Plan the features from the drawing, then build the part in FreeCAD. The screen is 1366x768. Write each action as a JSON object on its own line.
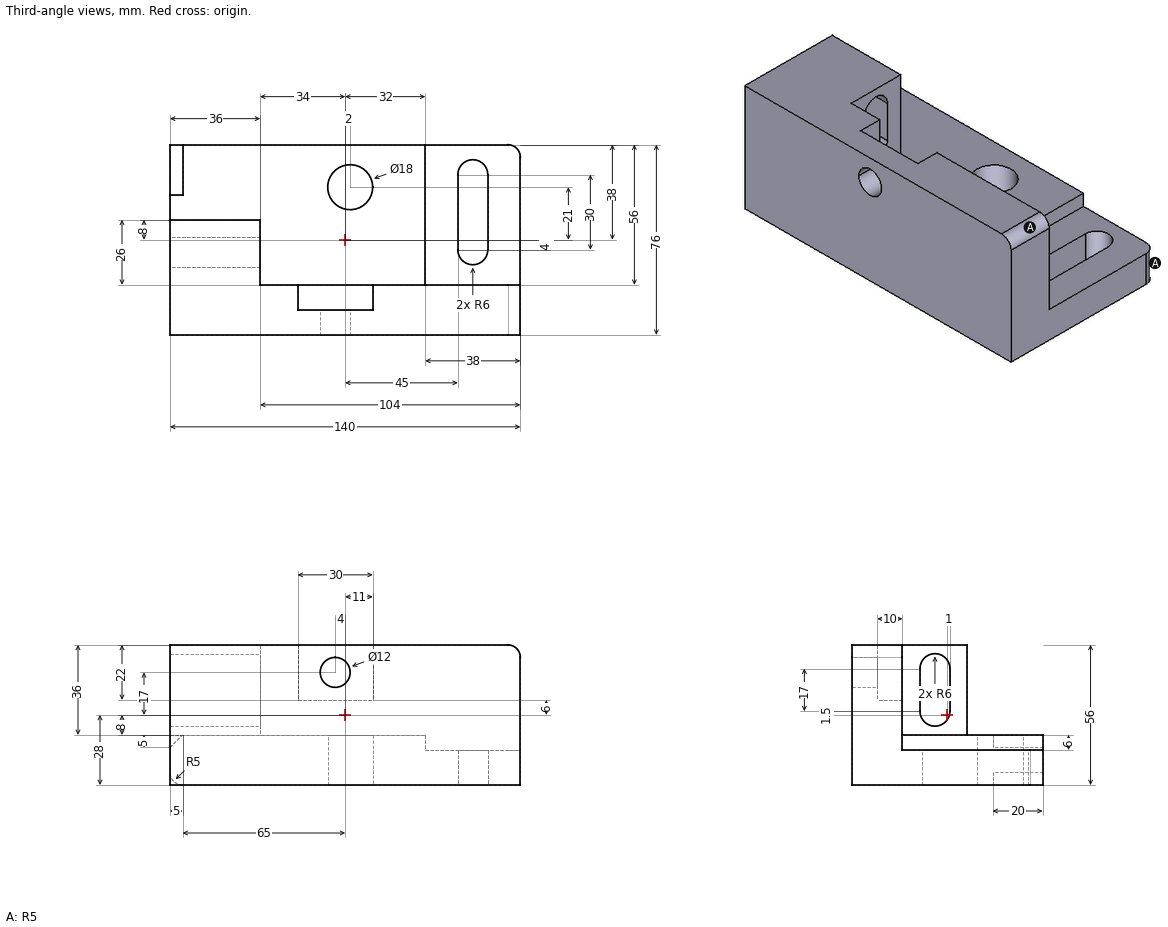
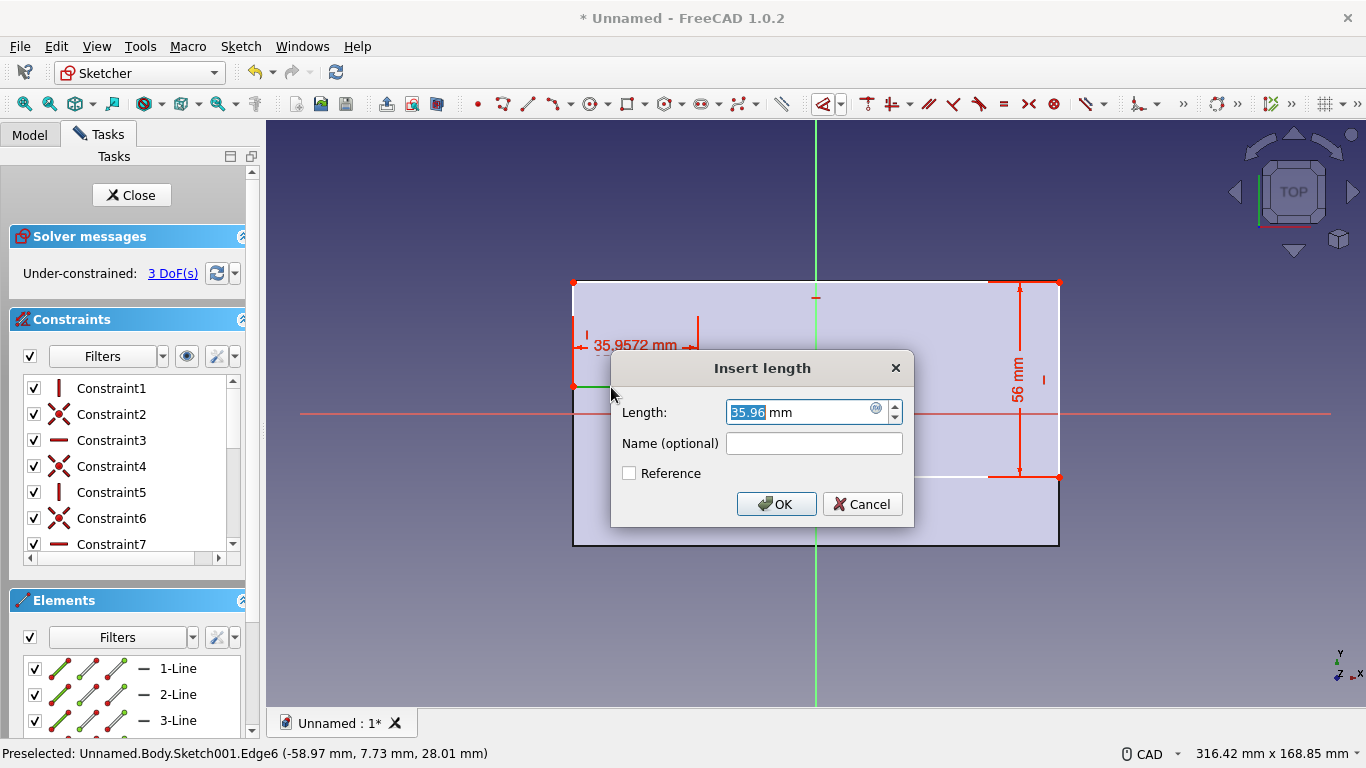
{"action": "type", "text": "36"}
{"action": "key", "text": "Return"}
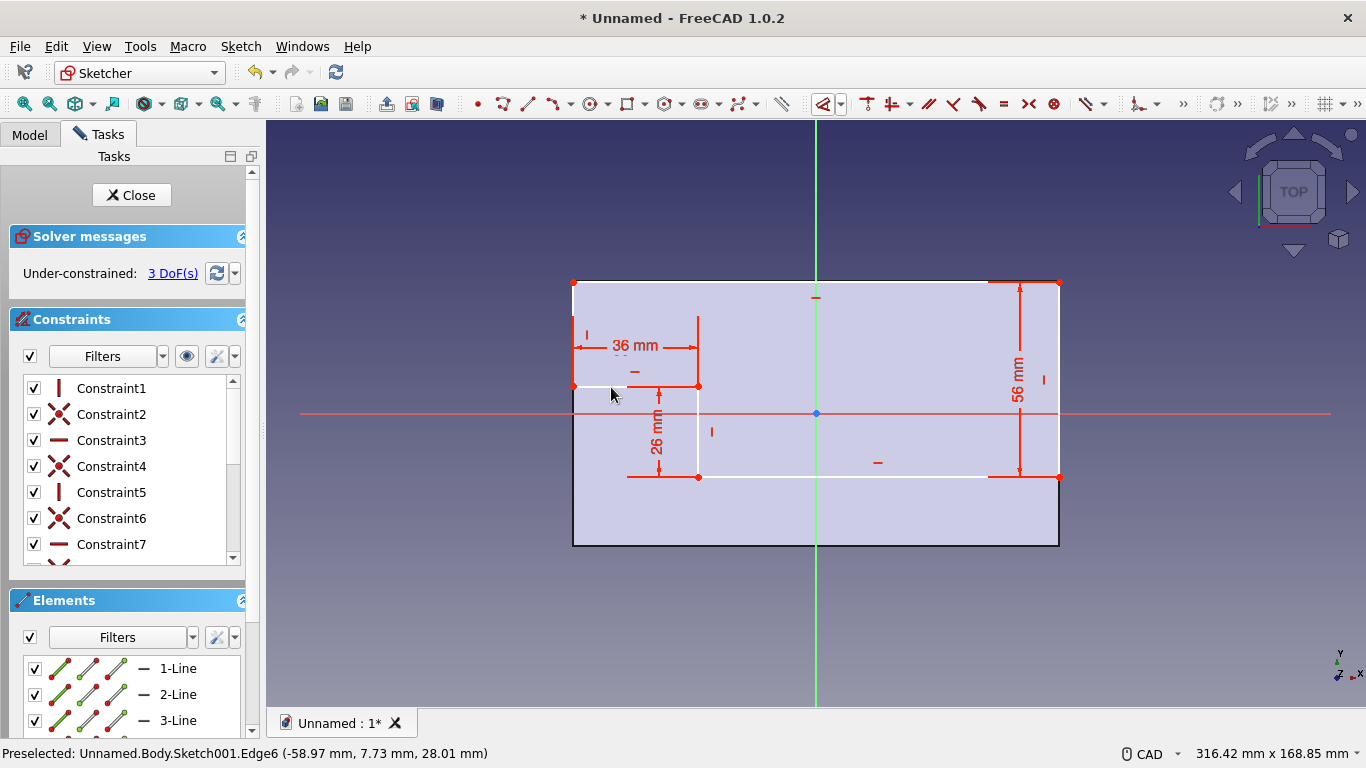
{"action": "scroll", "coordinate": [698, 387], "scroll_direction": "up", "scroll_amount": 2}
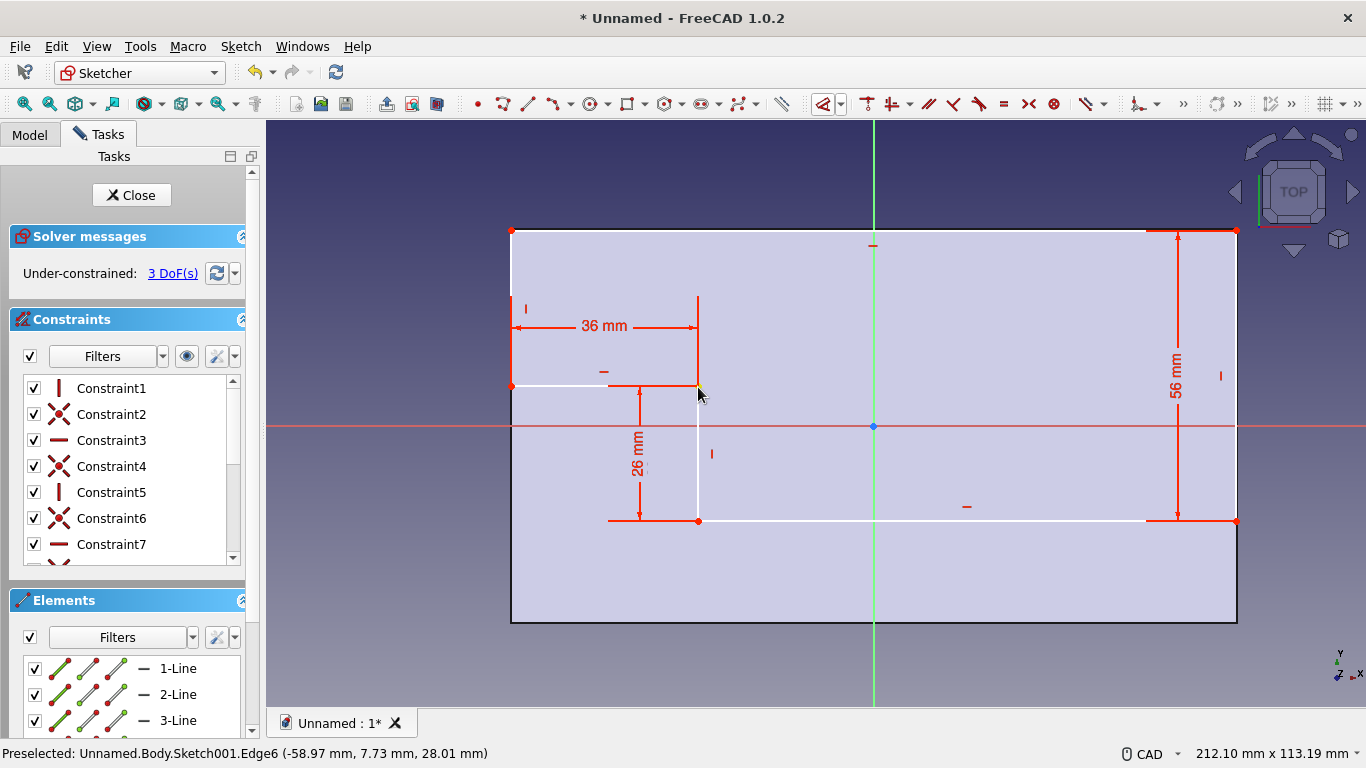
{"action": "left_click", "coordinate": [698, 386]}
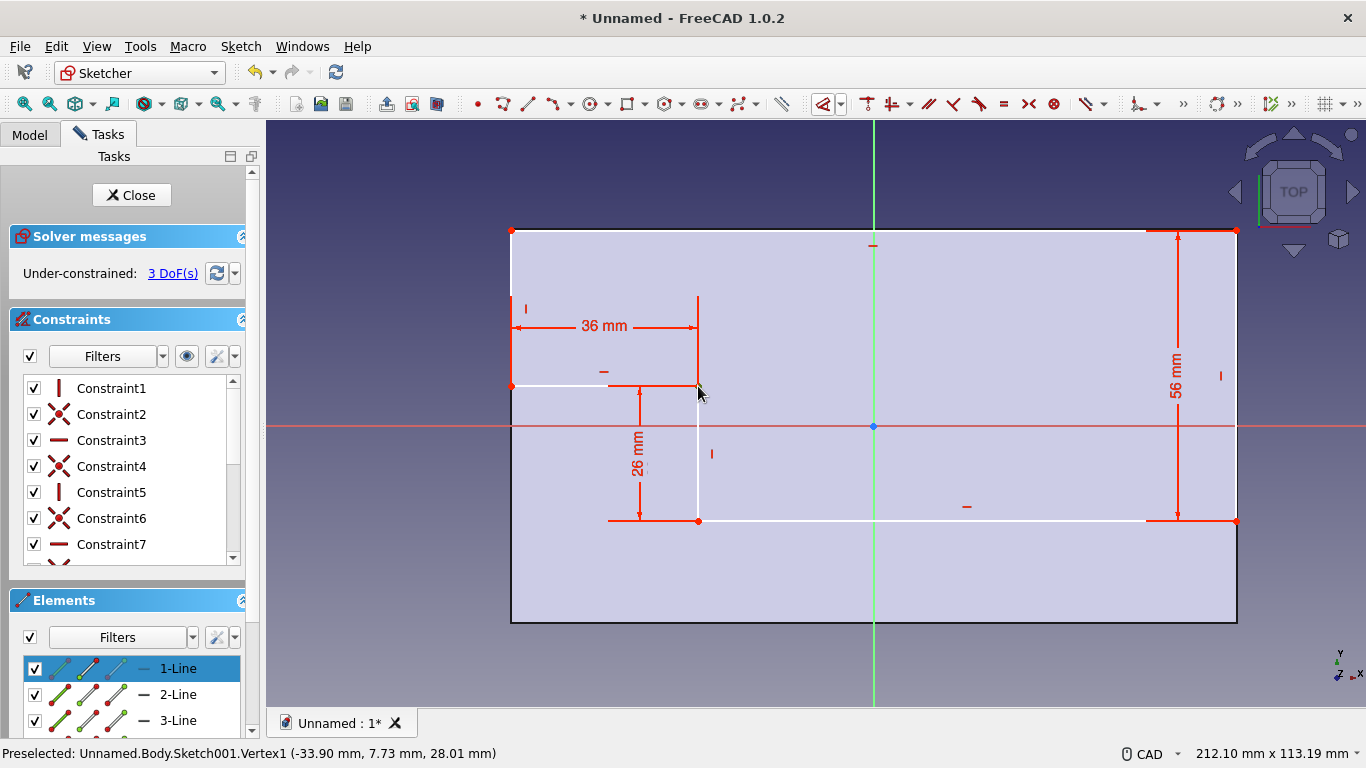
{"action": "left_click", "coordinate": [840, 104]}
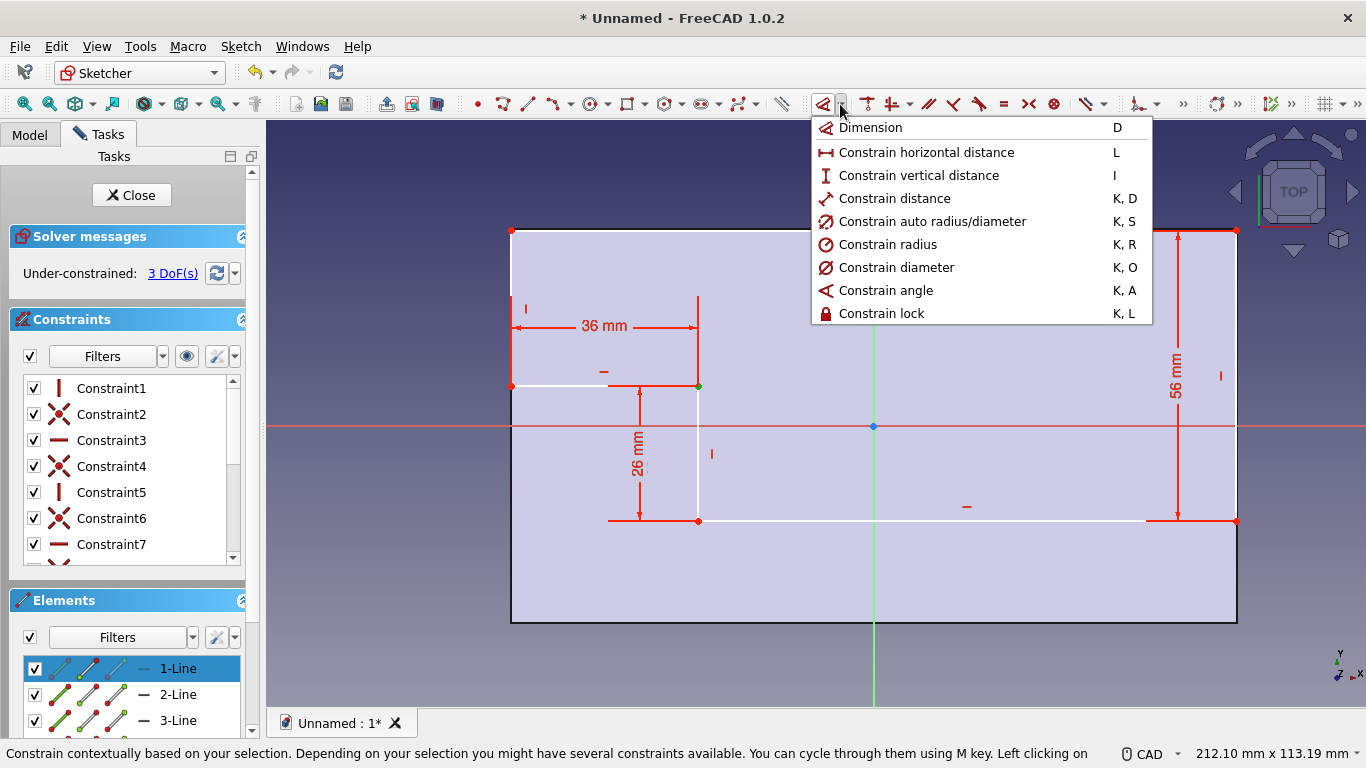
{"action": "left_click", "coordinate": [982, 176]}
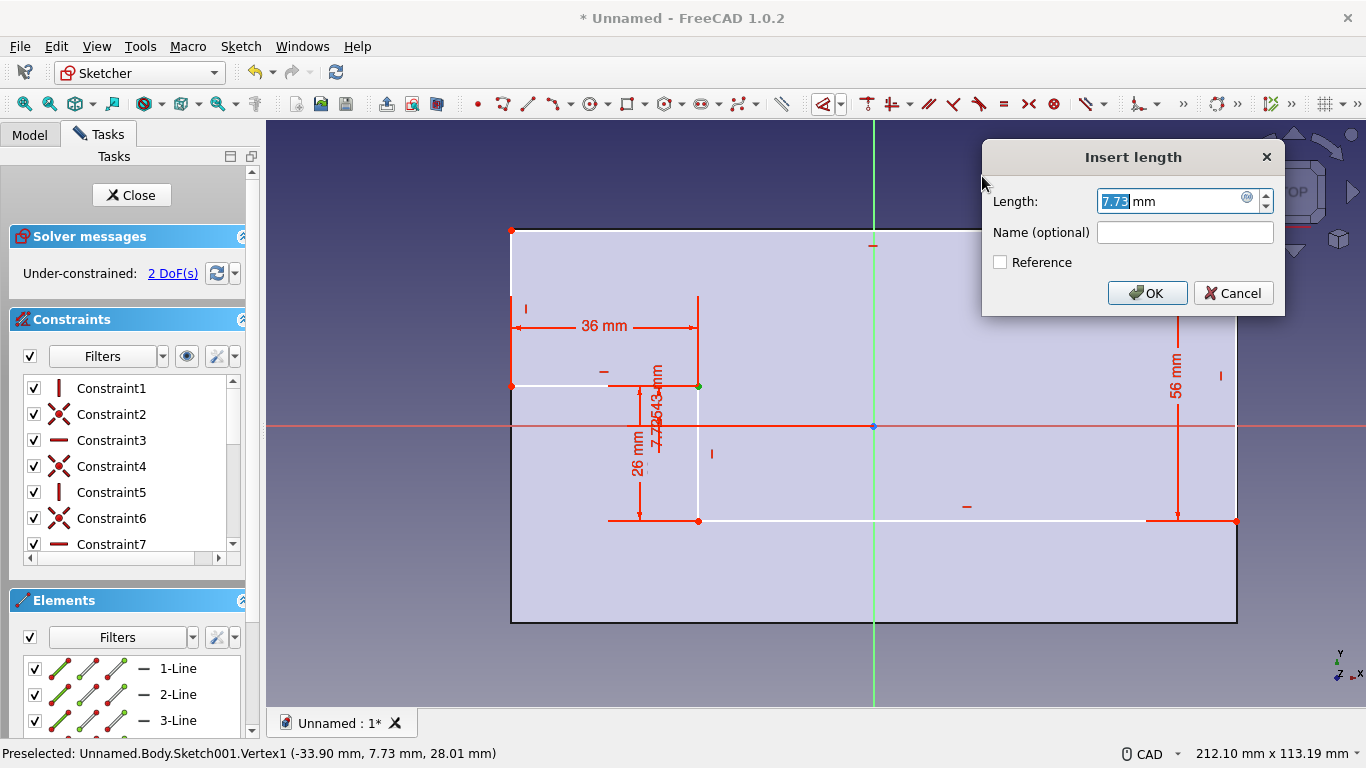
{"action": "type", "text": "8"}
{"action": "key", "text": "Return"}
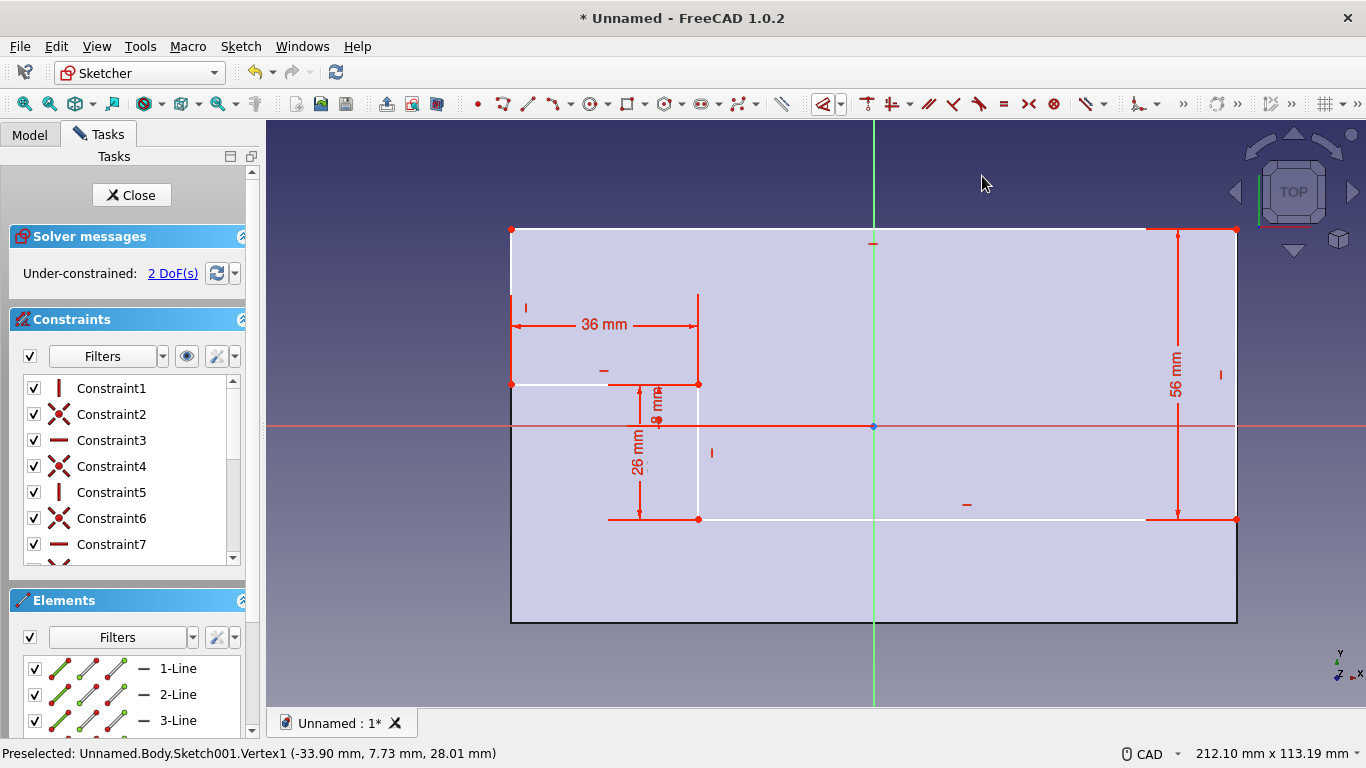
{"action": "left_click", "coordinate": [860, 520]}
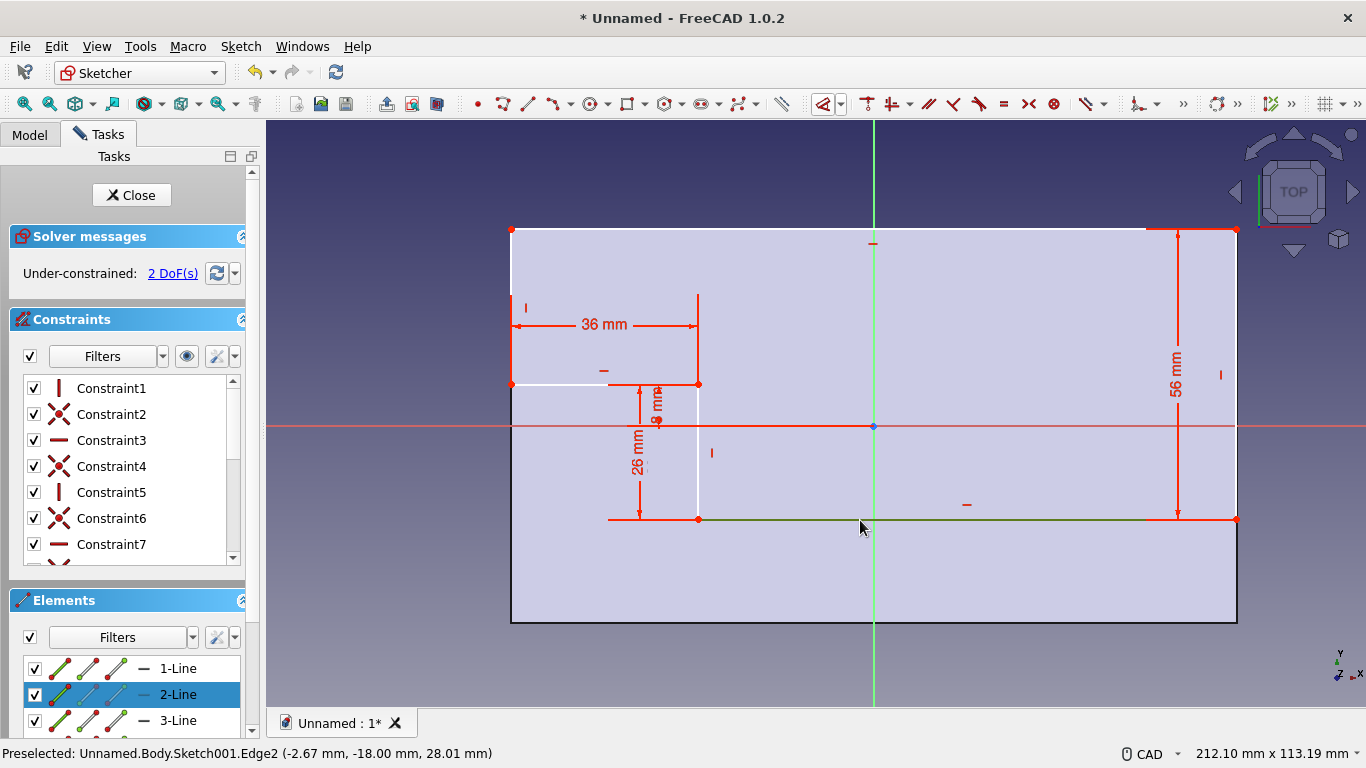
{"action": "left_click", "coordinate": [840, 104]}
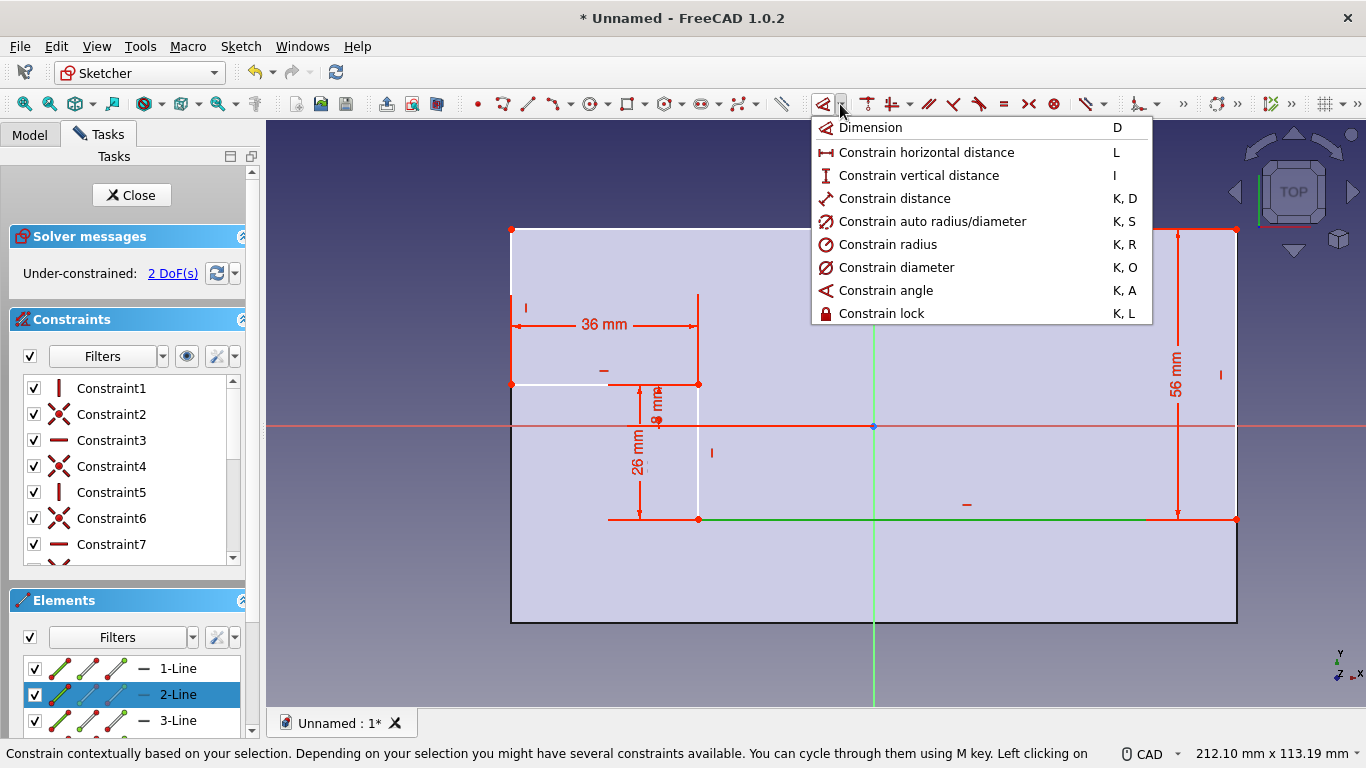
{"action": "left_click", "coordinate": [982, 152]}